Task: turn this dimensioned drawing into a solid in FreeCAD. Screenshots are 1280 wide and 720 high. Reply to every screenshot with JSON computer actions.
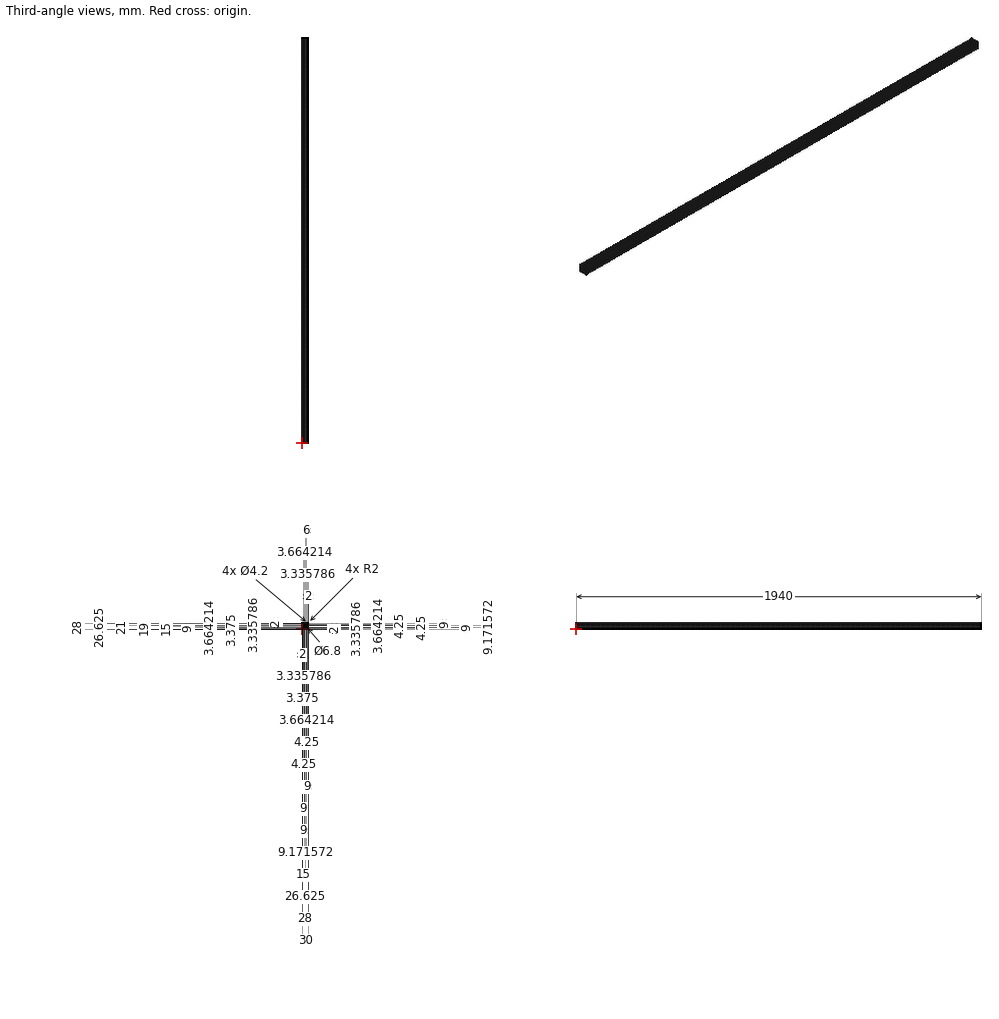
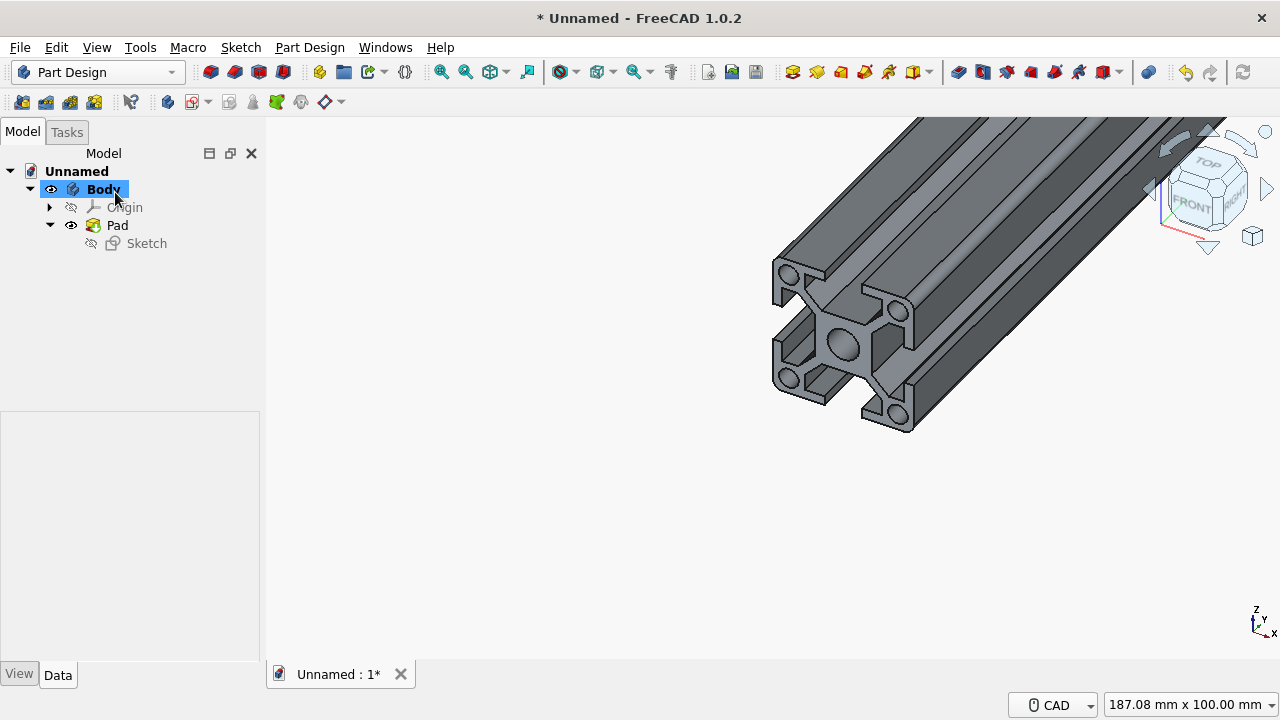
{"action": "key", "text": "0"}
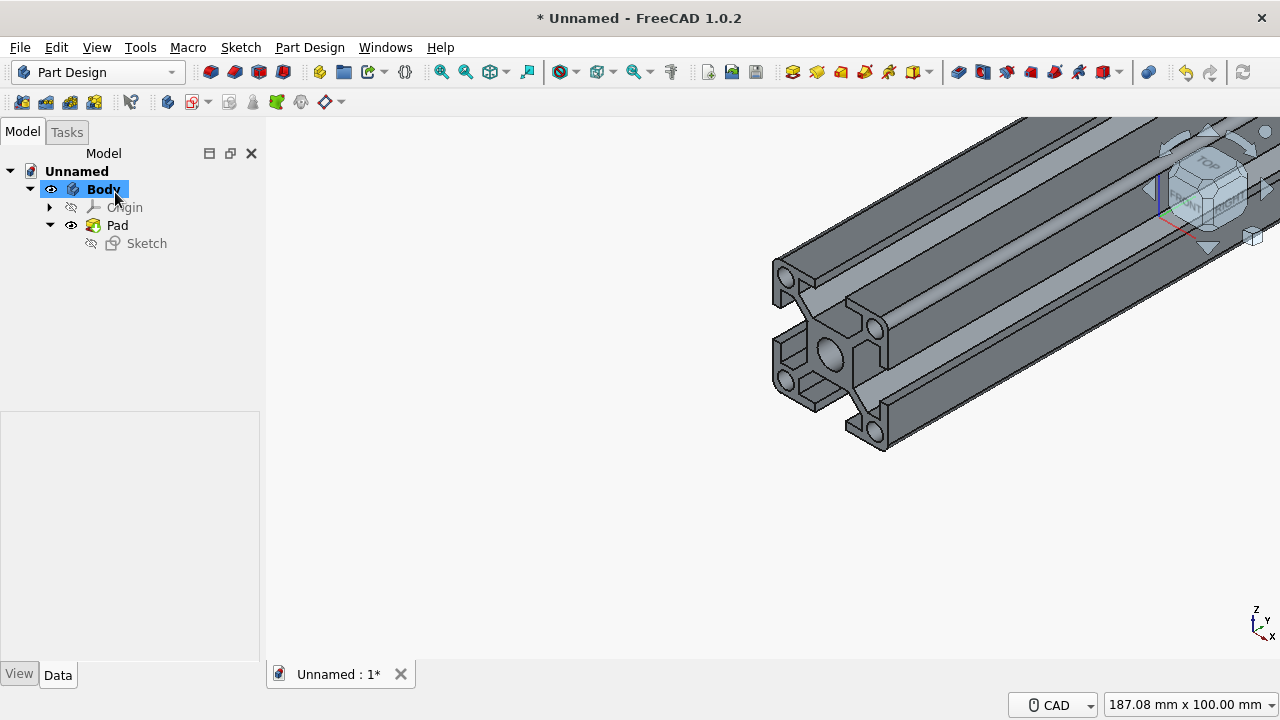
{"action": "left_click", "coordinate": [442, 72]}